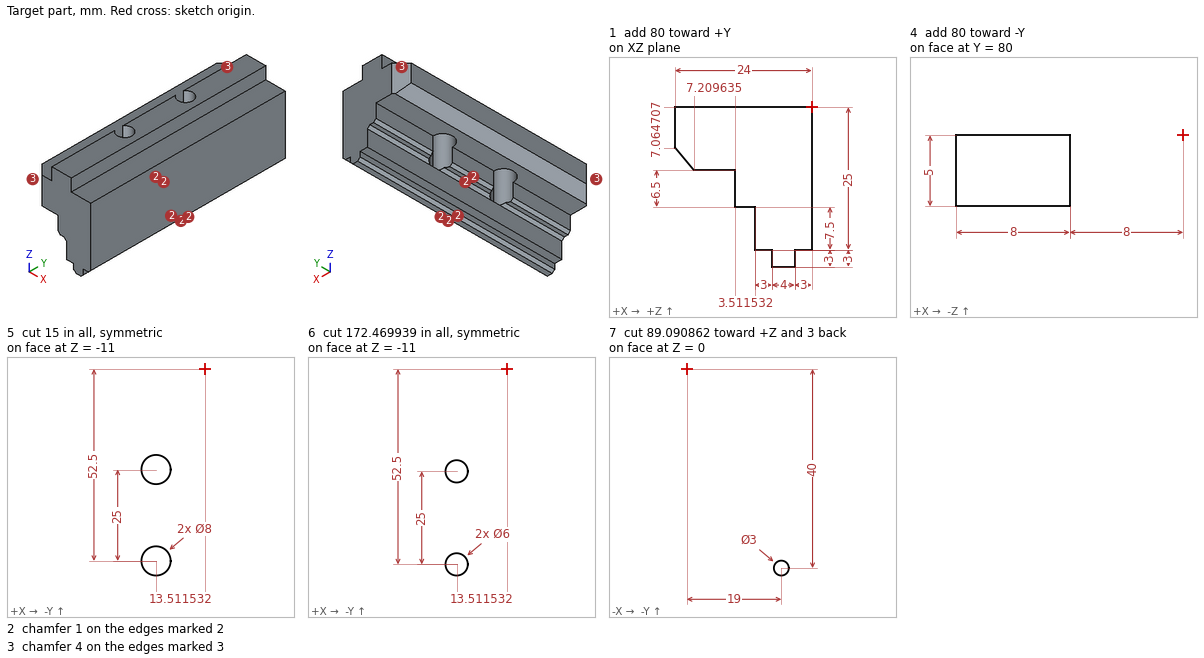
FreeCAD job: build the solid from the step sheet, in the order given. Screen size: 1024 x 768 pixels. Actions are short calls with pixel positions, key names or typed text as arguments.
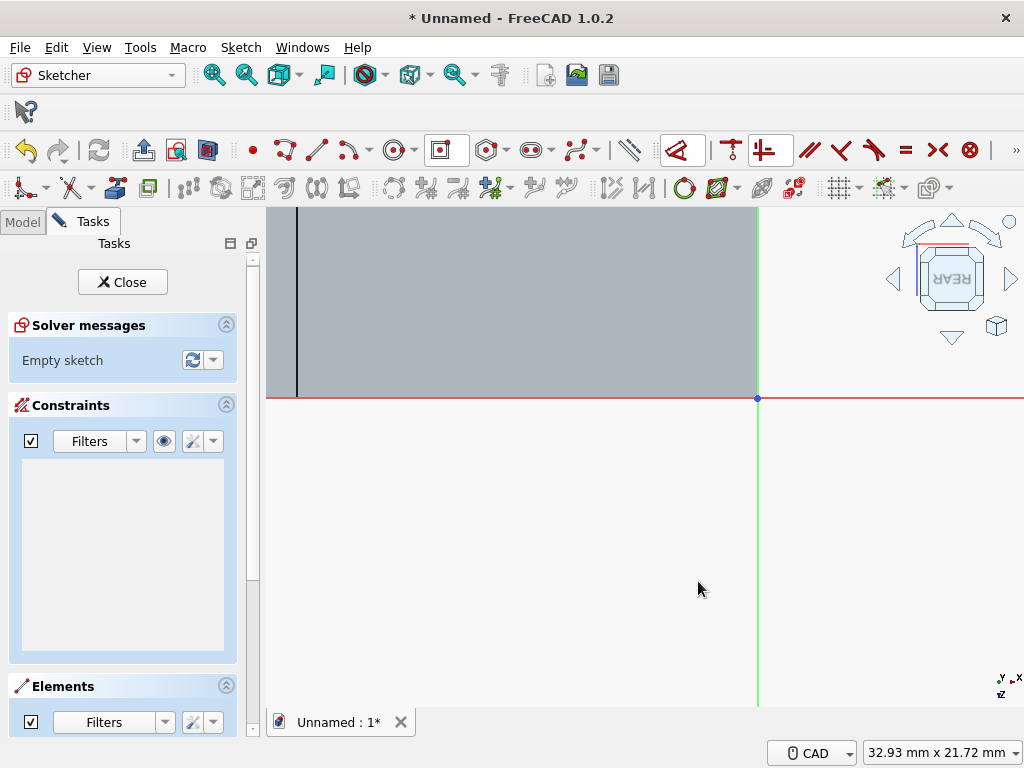
key(g)
key(r)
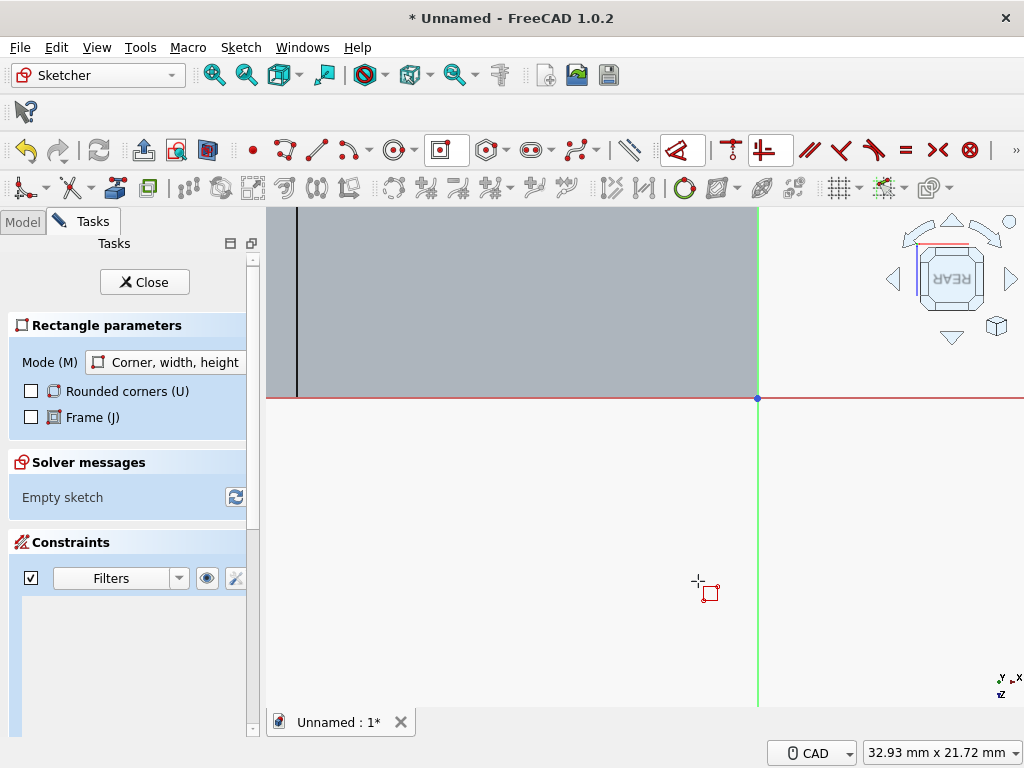
click(389, 398)
click(573, 513)
key(Escape)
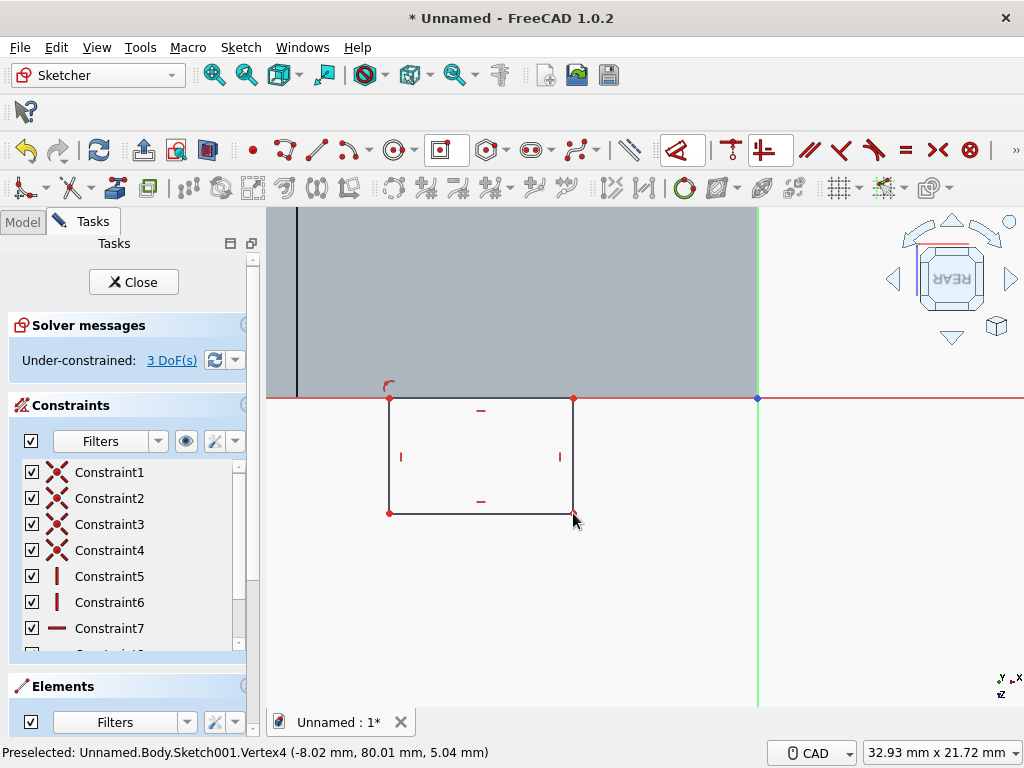
click(389, 433)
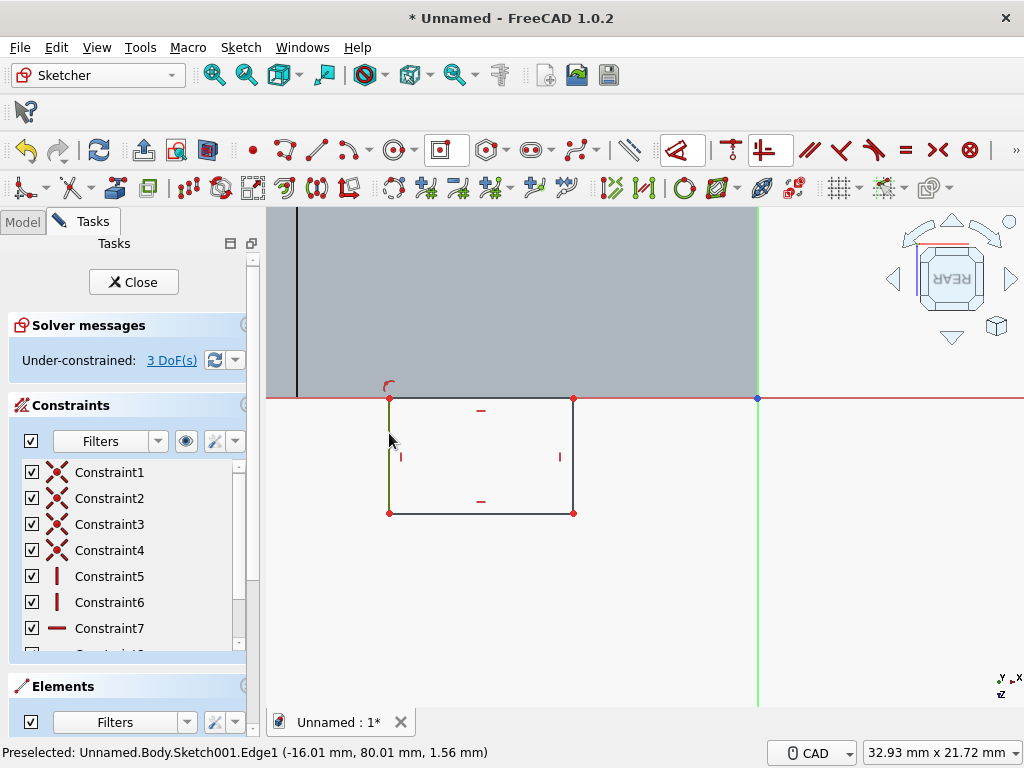
key(i)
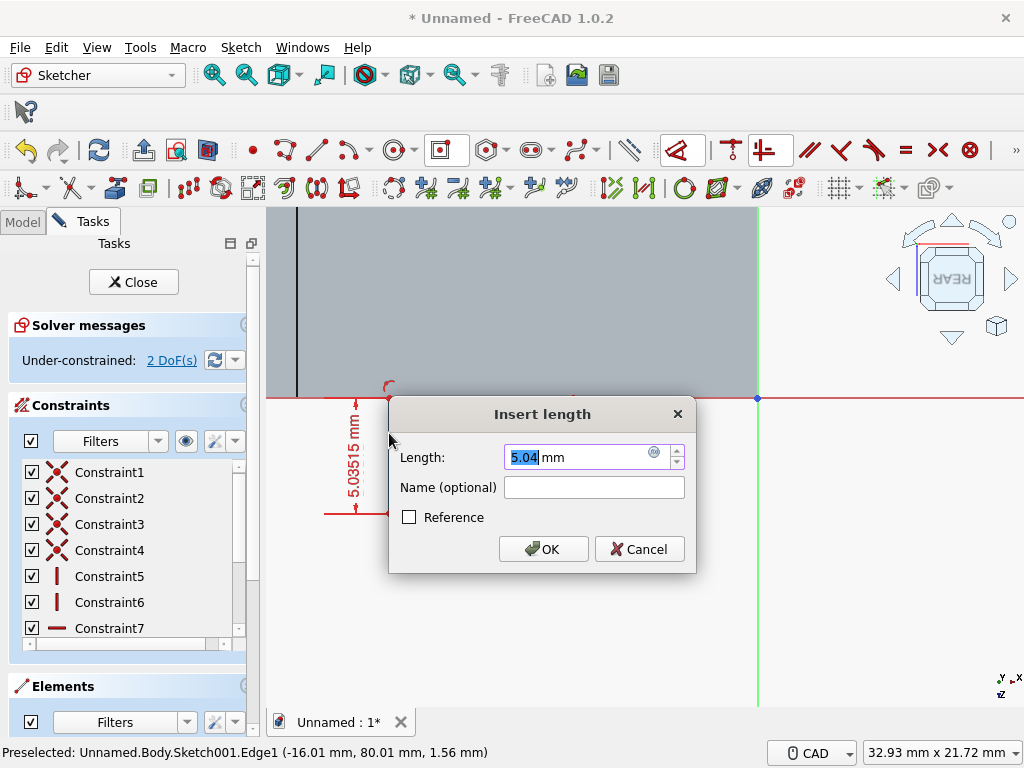
text(5)
key(Return)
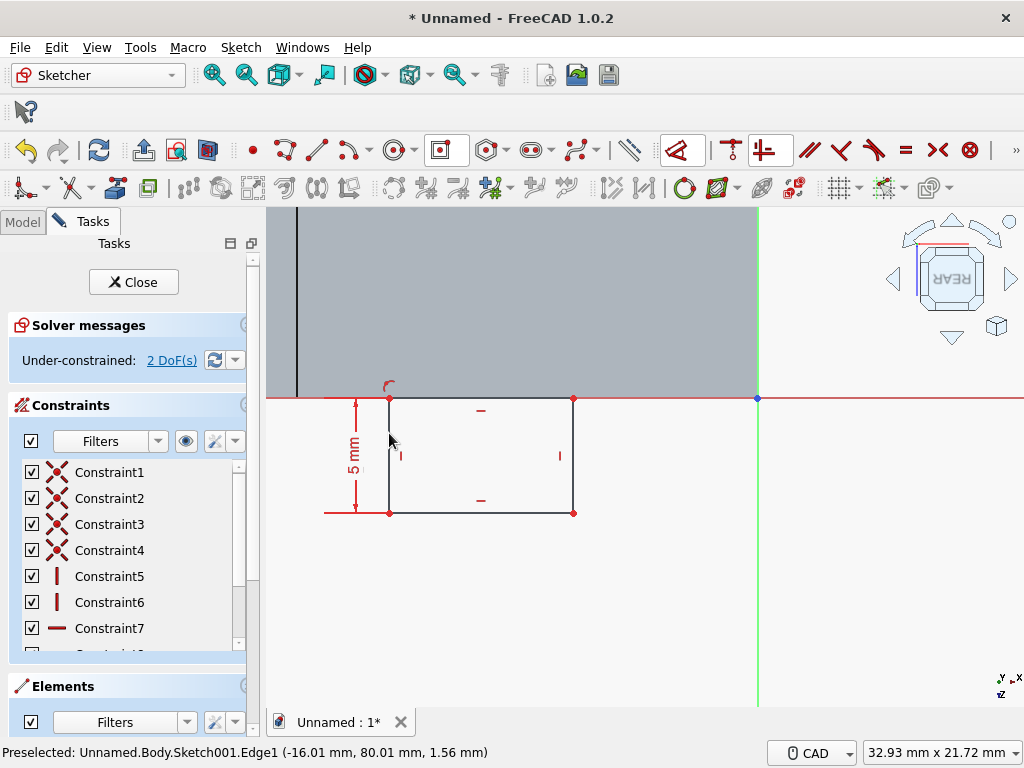
click(444, 513)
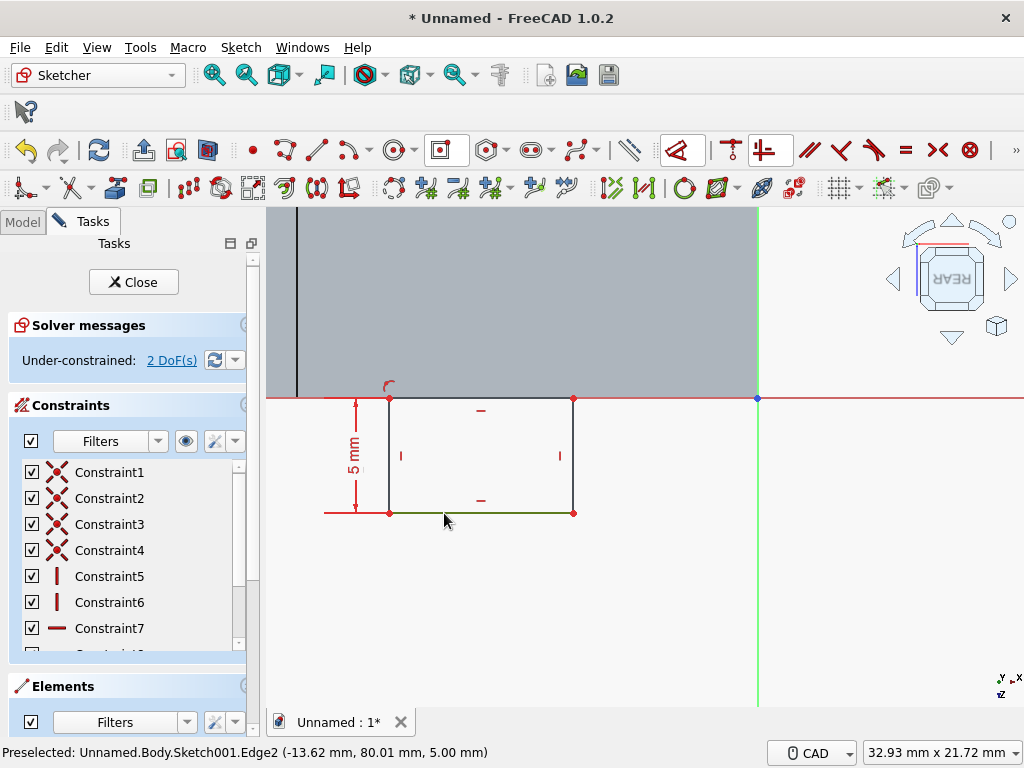
click(700, 150)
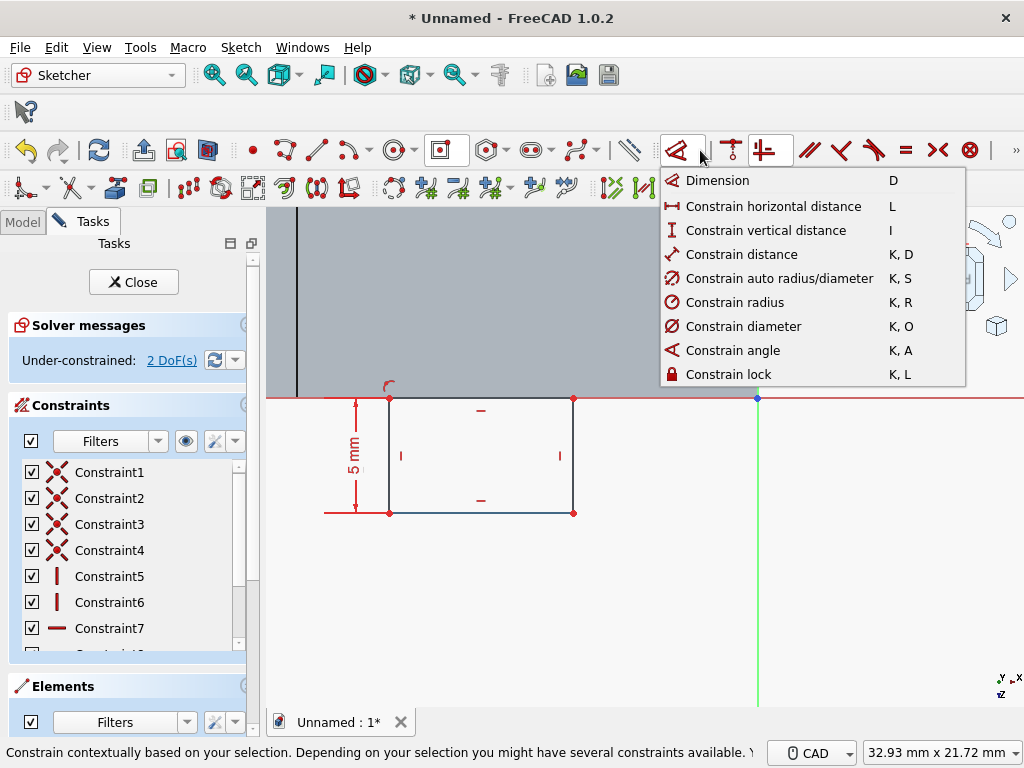
click(813, 206)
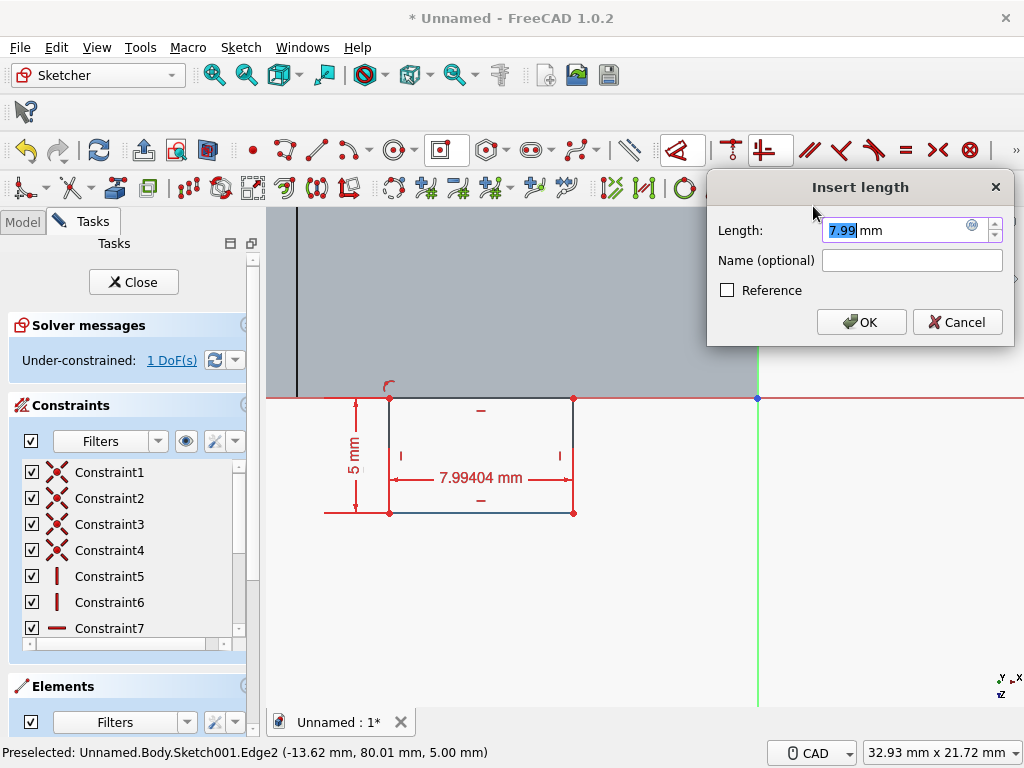
text(8)
key(Return)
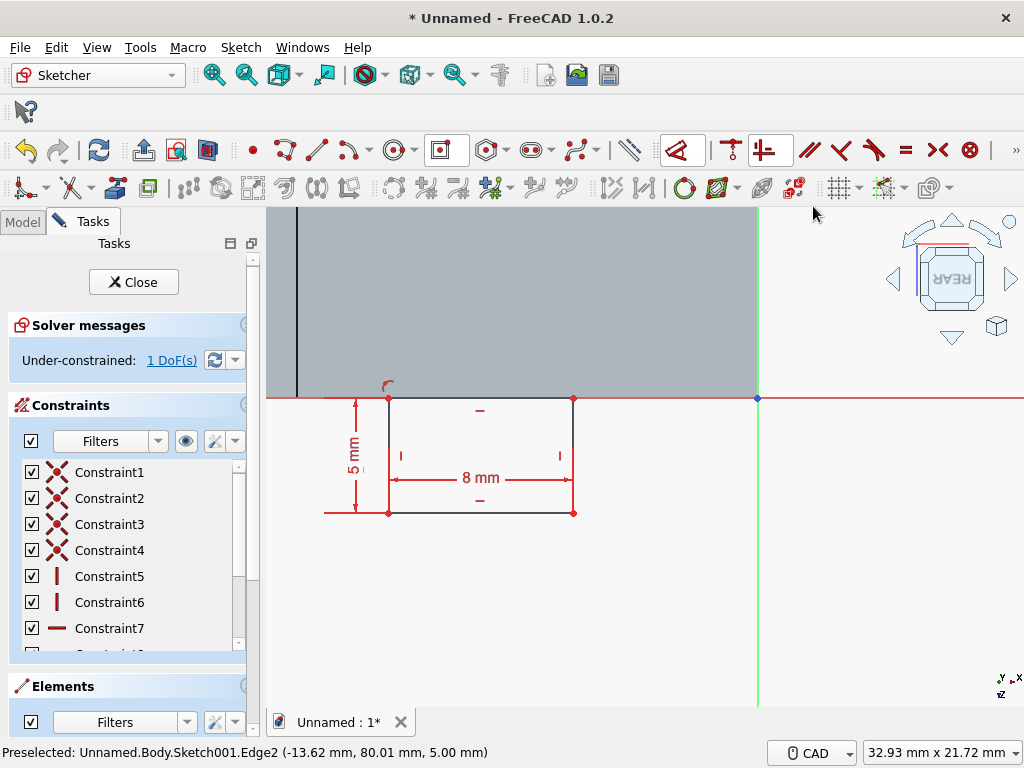
click(573, 513)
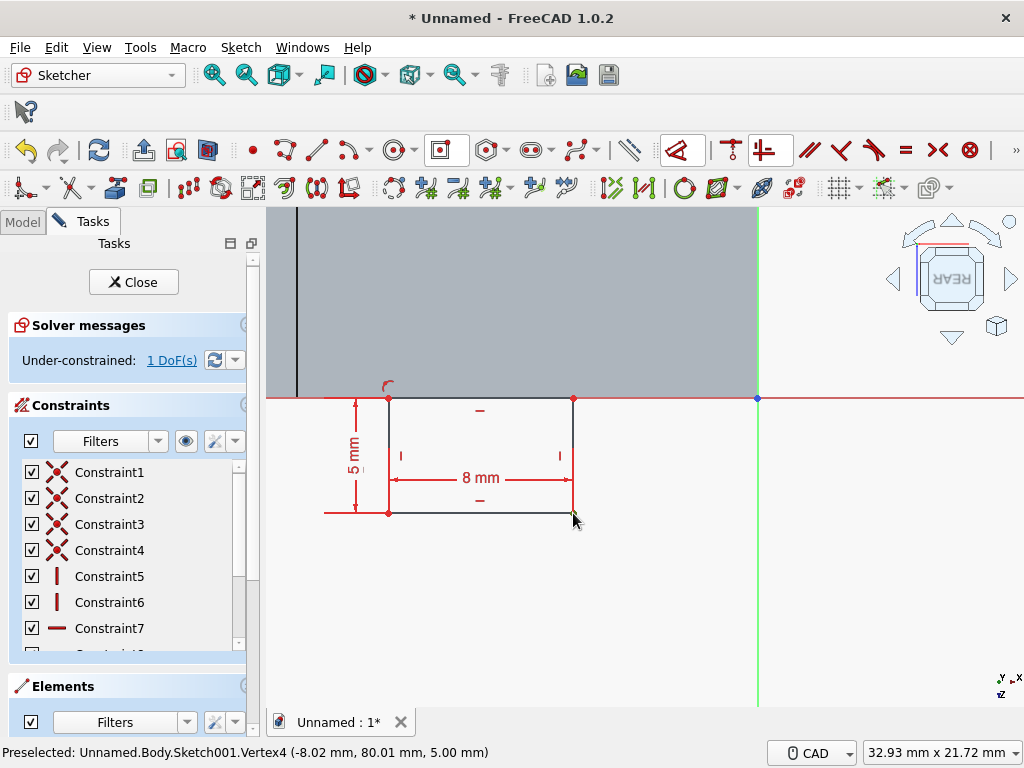
key(l)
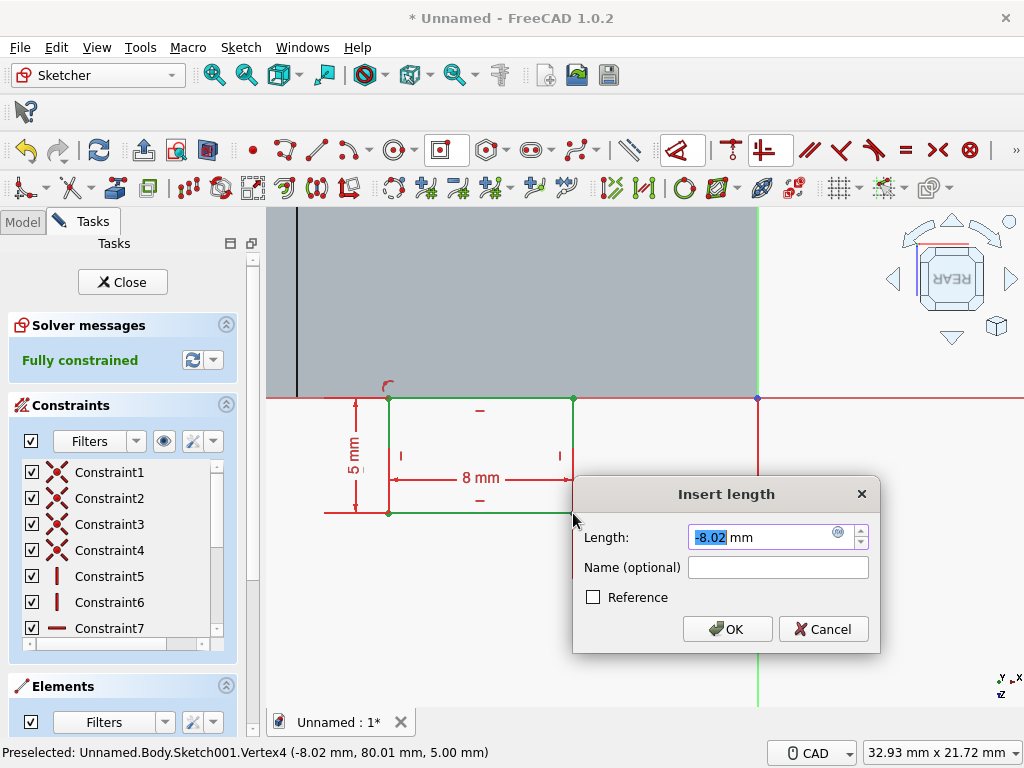
text(-8)
key(Return)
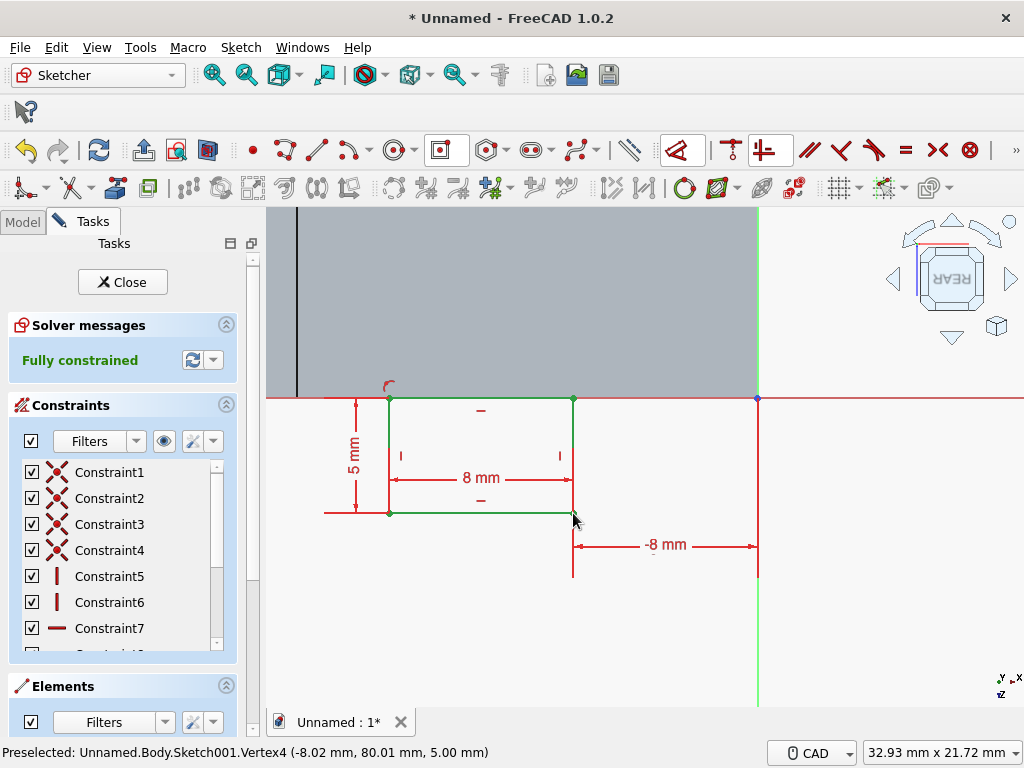
click(123, 282)